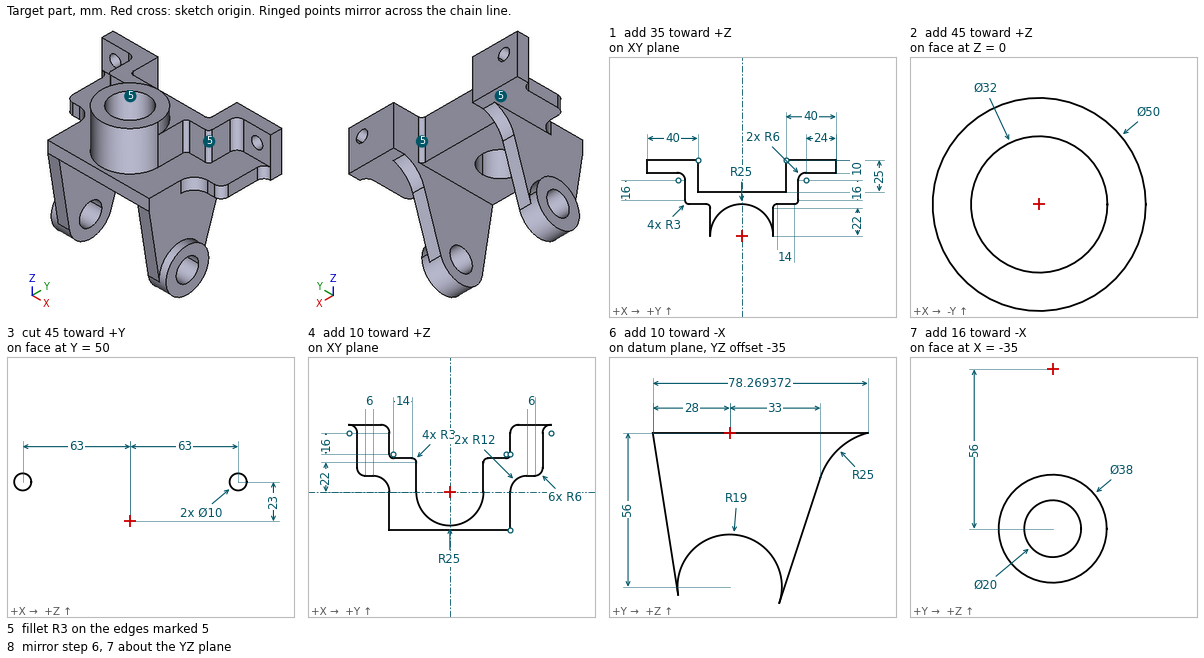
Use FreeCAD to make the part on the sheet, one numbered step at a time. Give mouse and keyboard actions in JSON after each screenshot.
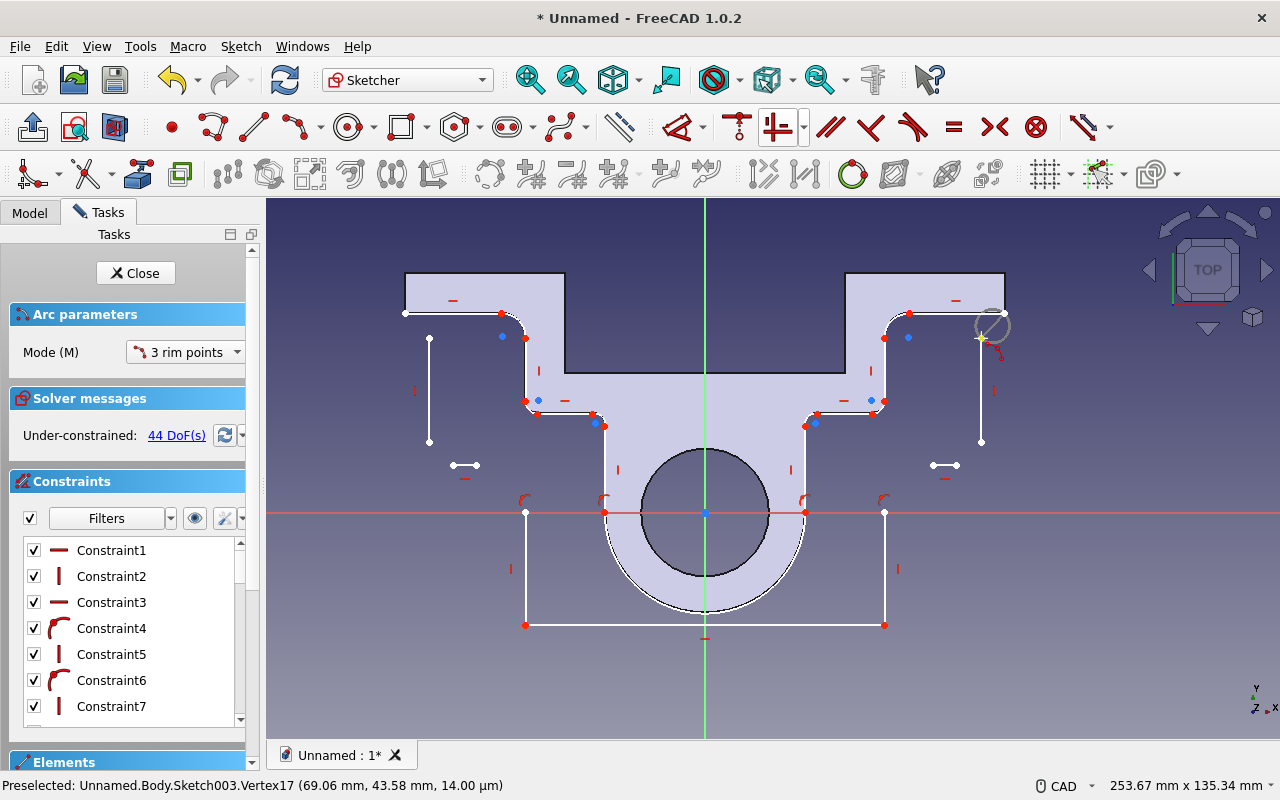
{"action": "scroll", "coordinate": [988, 320], "scroll_direction": "up", "scroll_amount": 5}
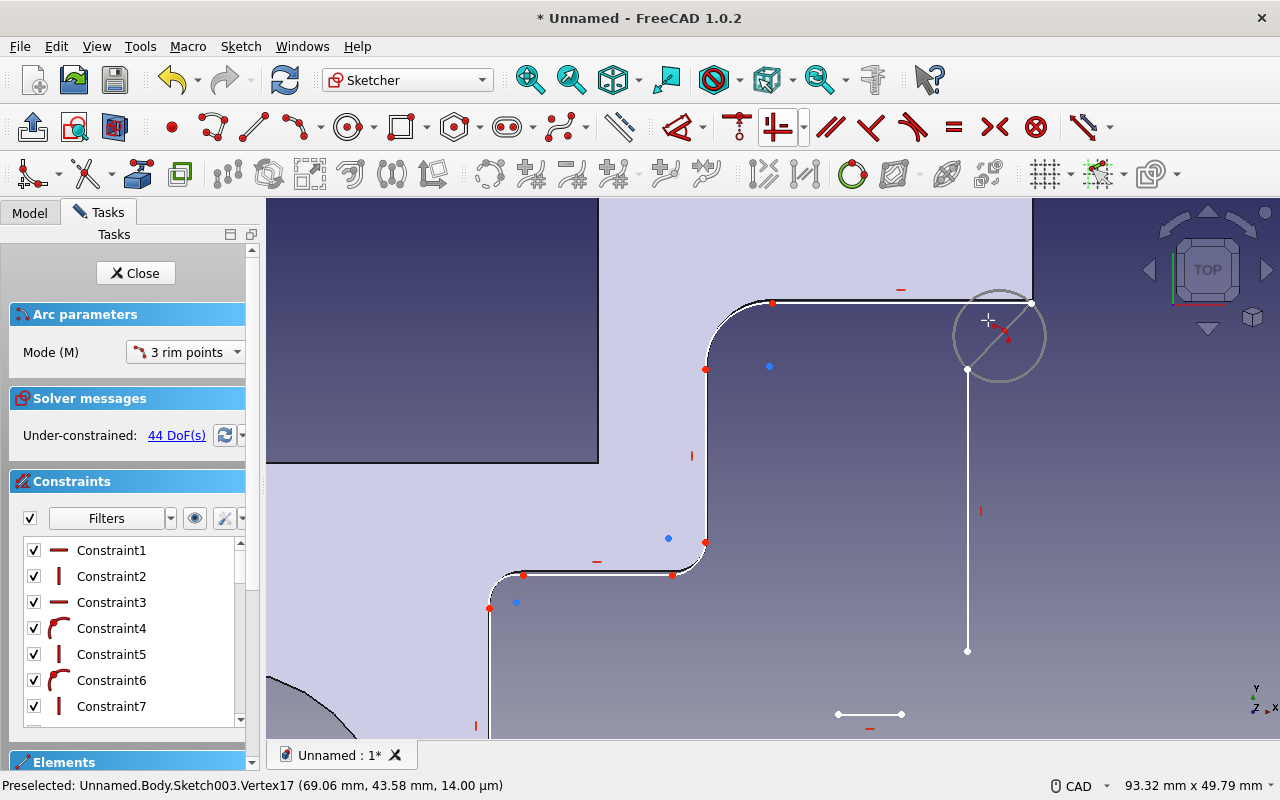
{"action": "left_click", "coordinate": [986, 319]}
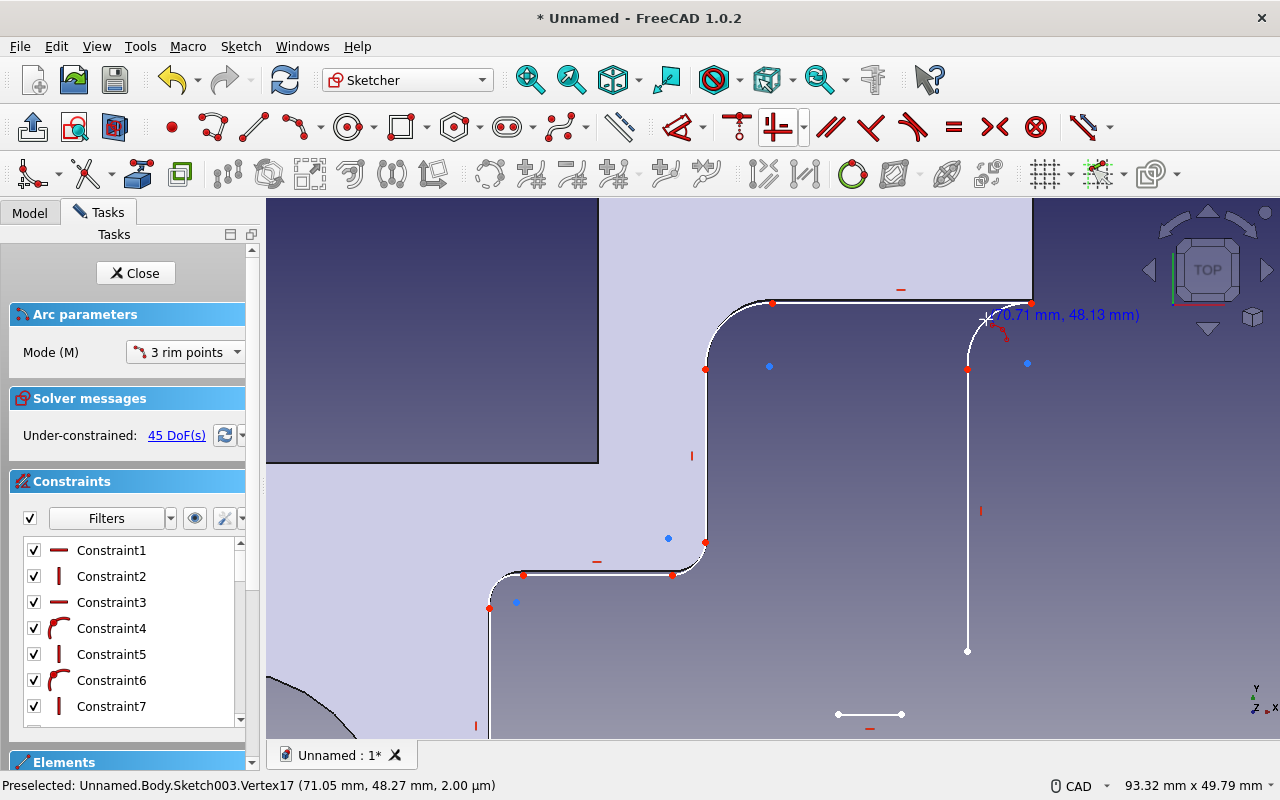
{"action": "left_click", "coordinate": [968, 652]}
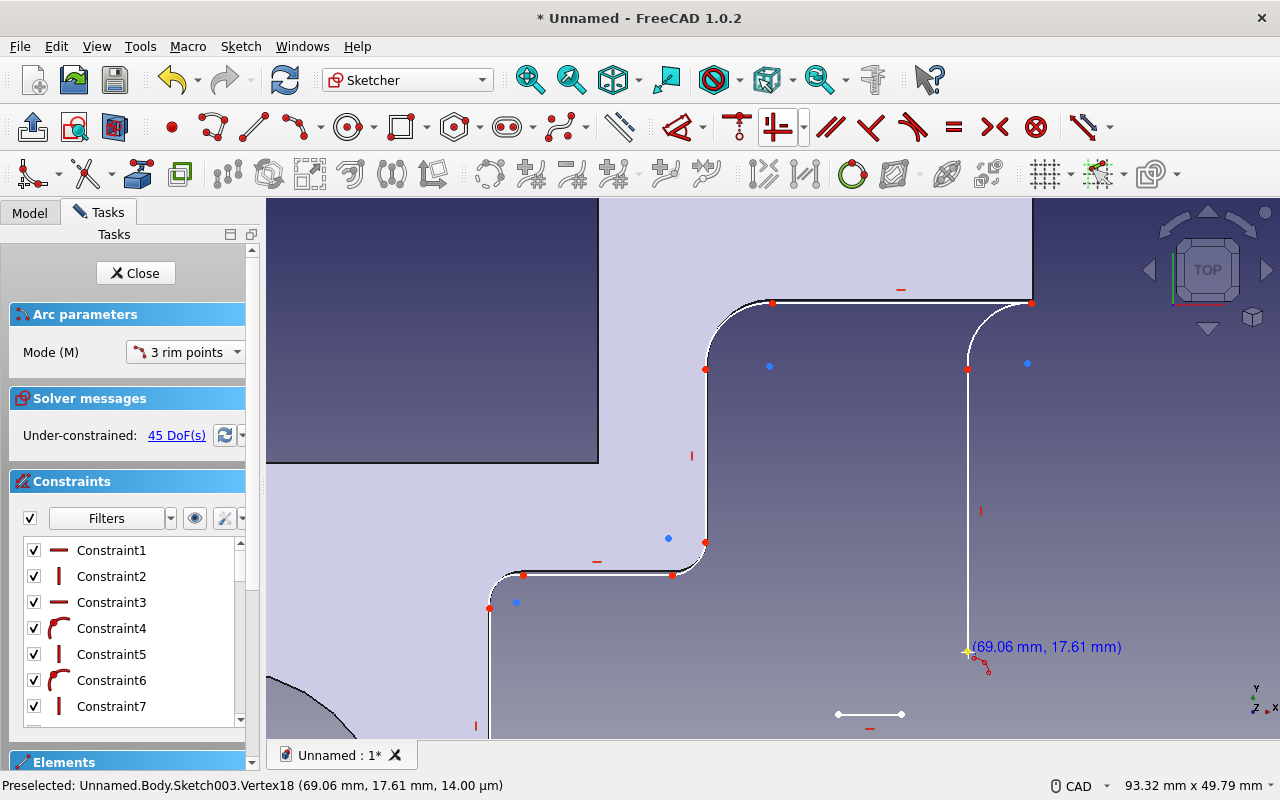
{"action": "scroll", "coordinate": [988, 320], "scroll_direction": "down", "scroll_amount": 5}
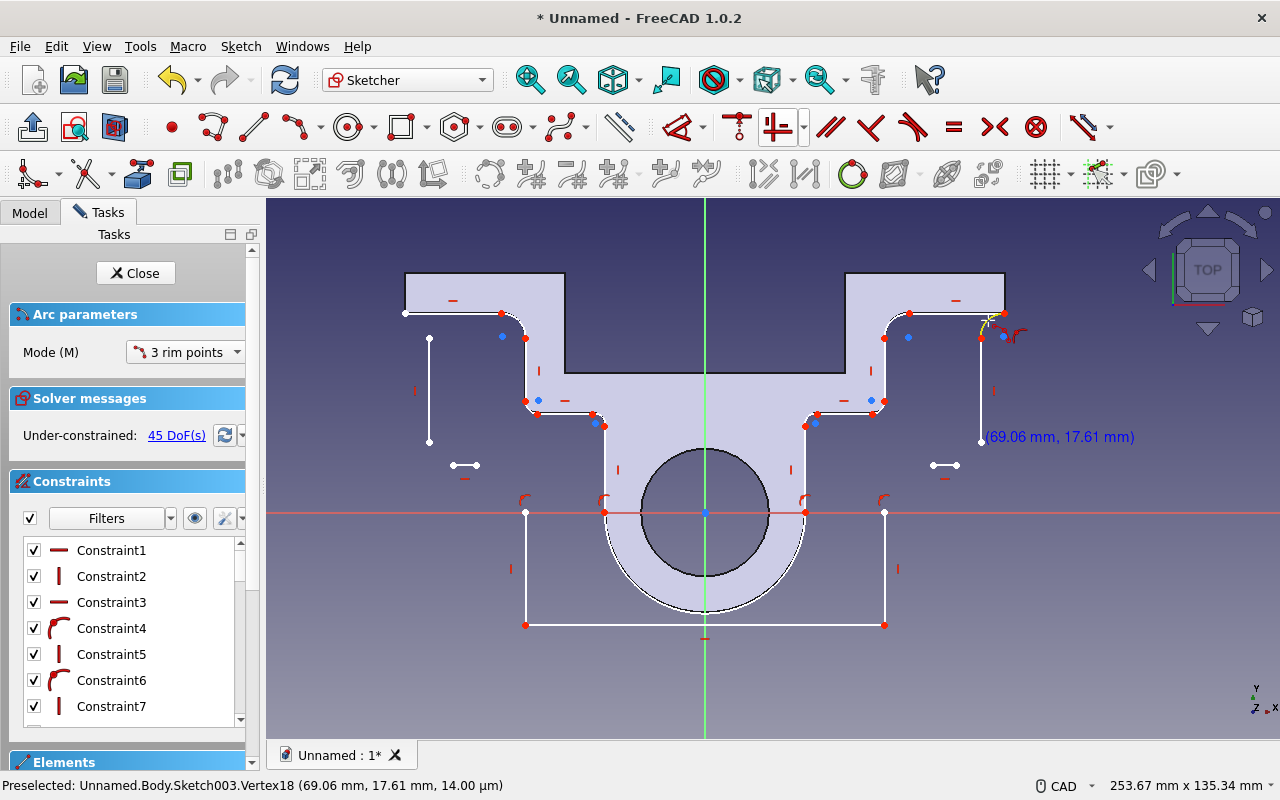
{"action": "scroll", "coordinate": [957, 465], "scroll_direction": "up", "scroll_amount": 2}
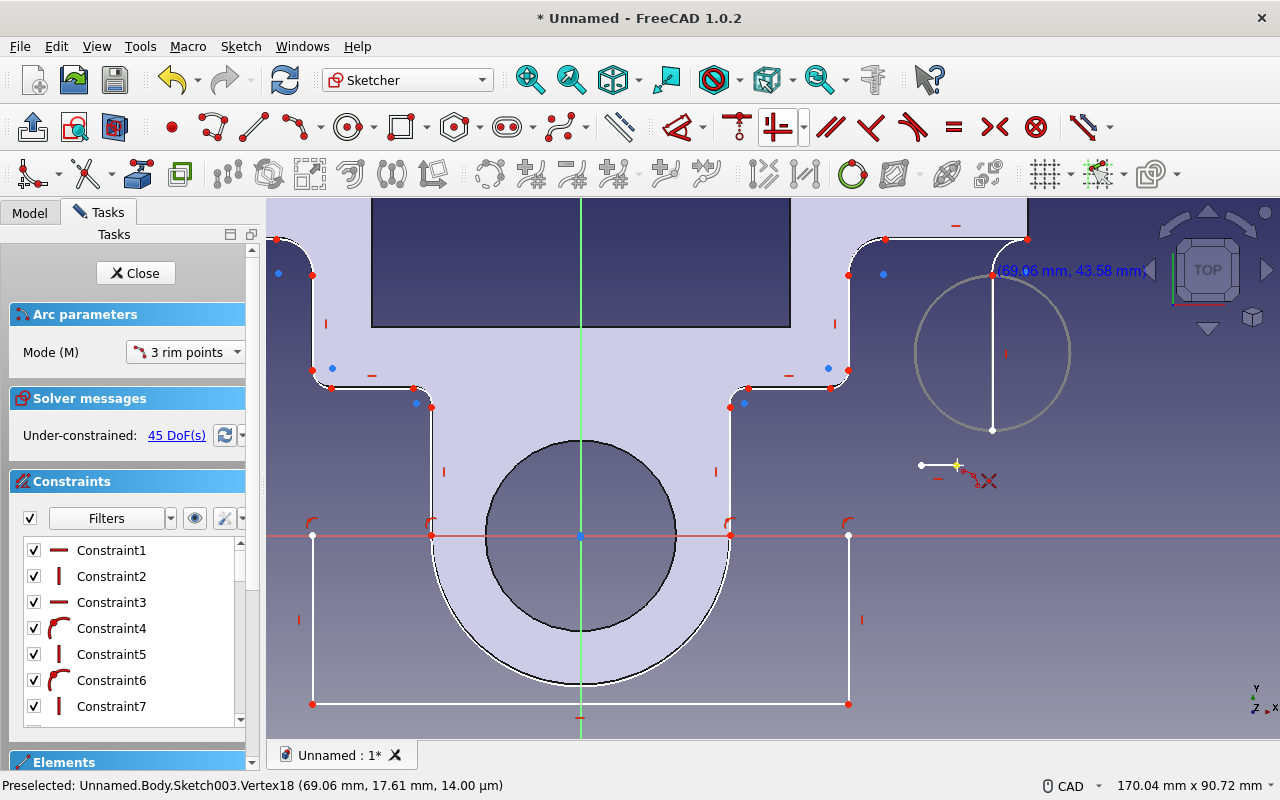
{"action": "left_click", "coordinate": [956, 465]}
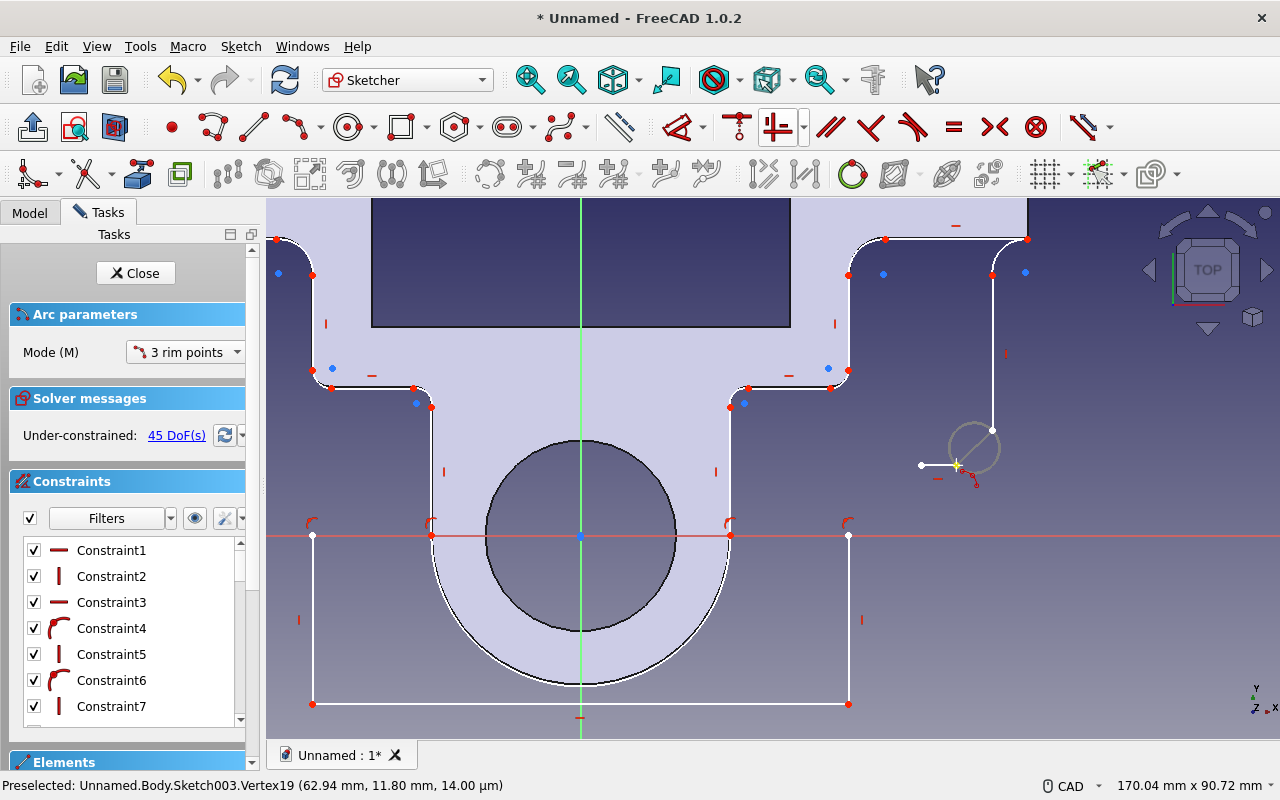
{"action": "scroll", "coordinate": [982, 454], "scroll_direction": "up", "scroll_amount": 3}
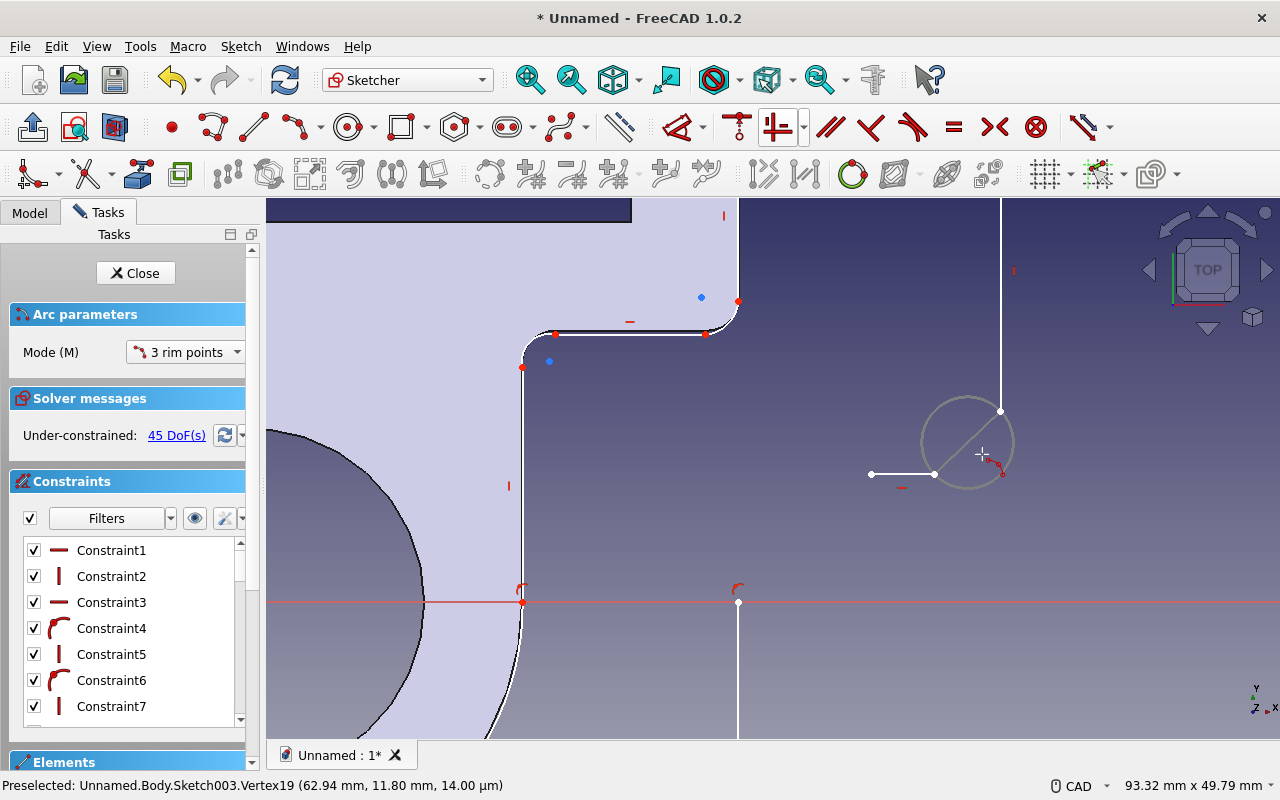
{"action": "left_click", "coordinate": [981, 453]}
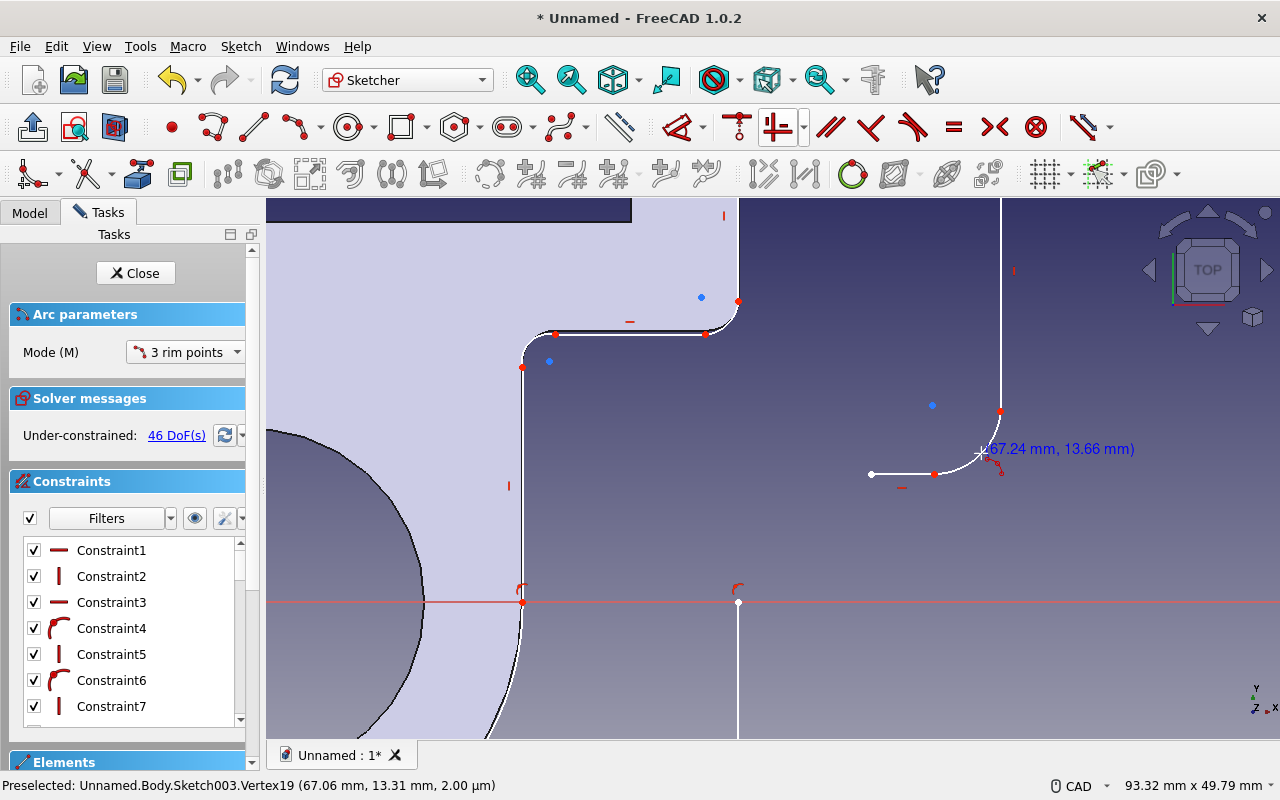
{"action": "left_click", "coordinate": [871, 474]}
{"action": "left_click", "coordinate": [738, 602]}
{"action": "left_click", "coordinate": [778, 510]}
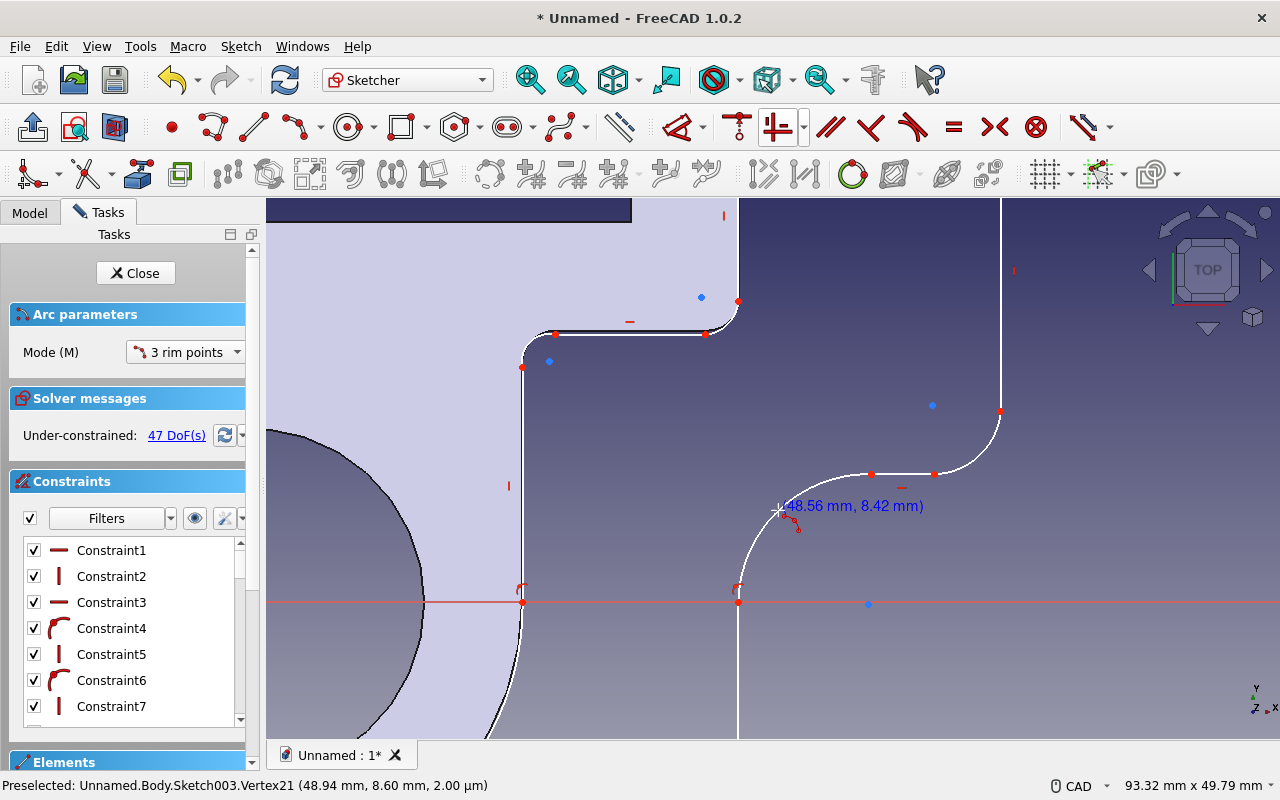
{"action": "scroll", "coordinate": [969, 460], "scroll_direction": "down", "scroll_amount": 5}